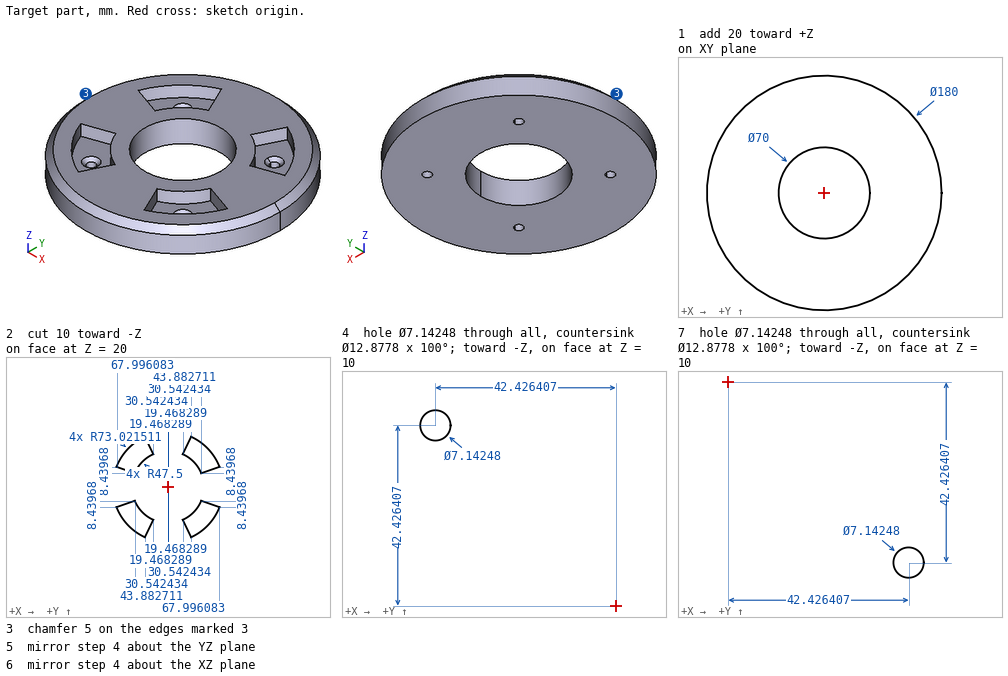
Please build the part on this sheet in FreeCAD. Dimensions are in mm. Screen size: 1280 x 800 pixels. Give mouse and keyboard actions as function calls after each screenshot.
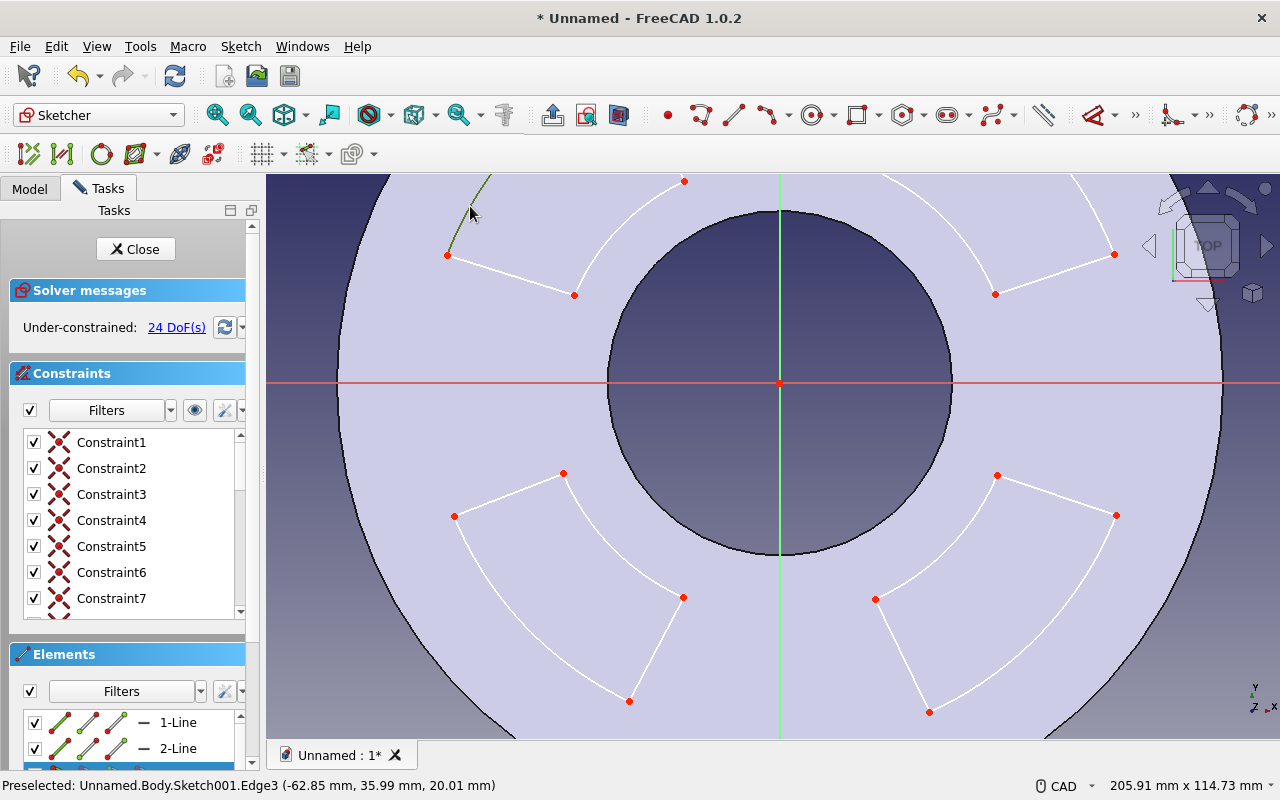
click(1091, 205)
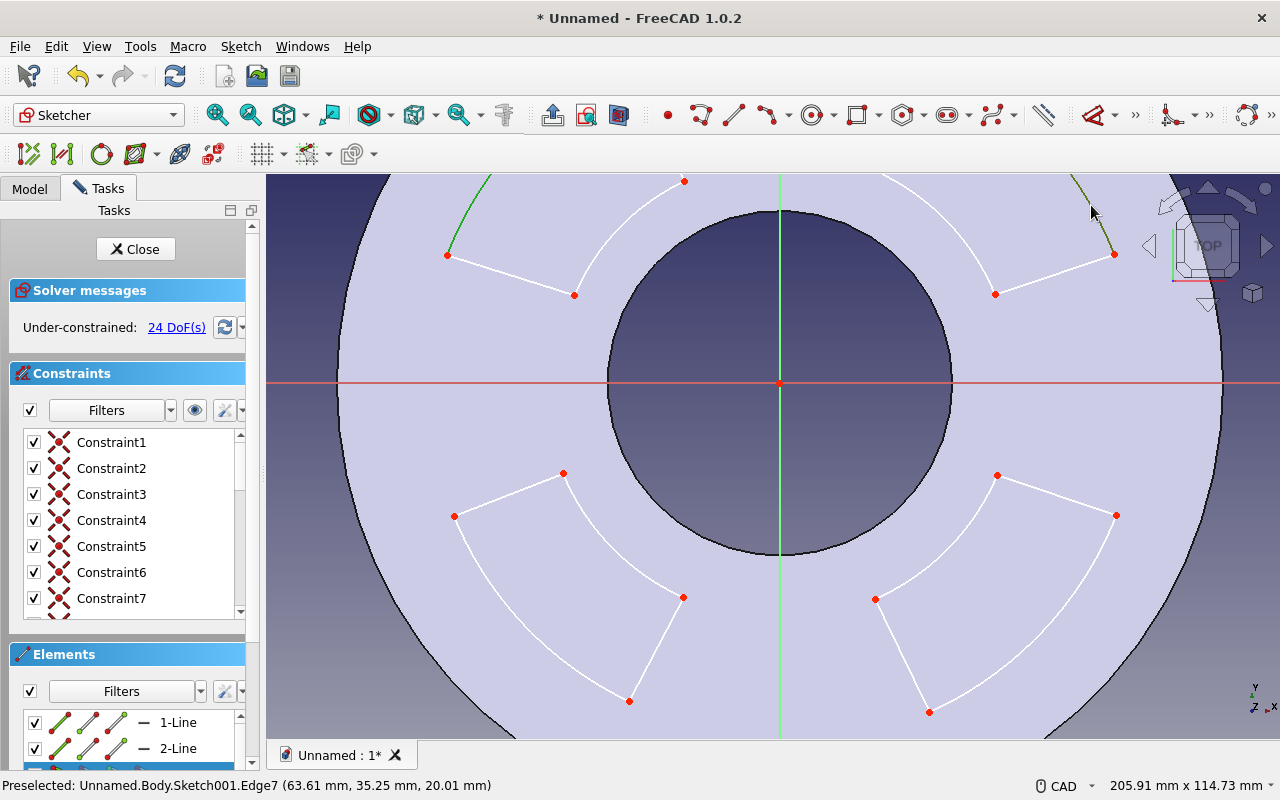
click(1001, 669)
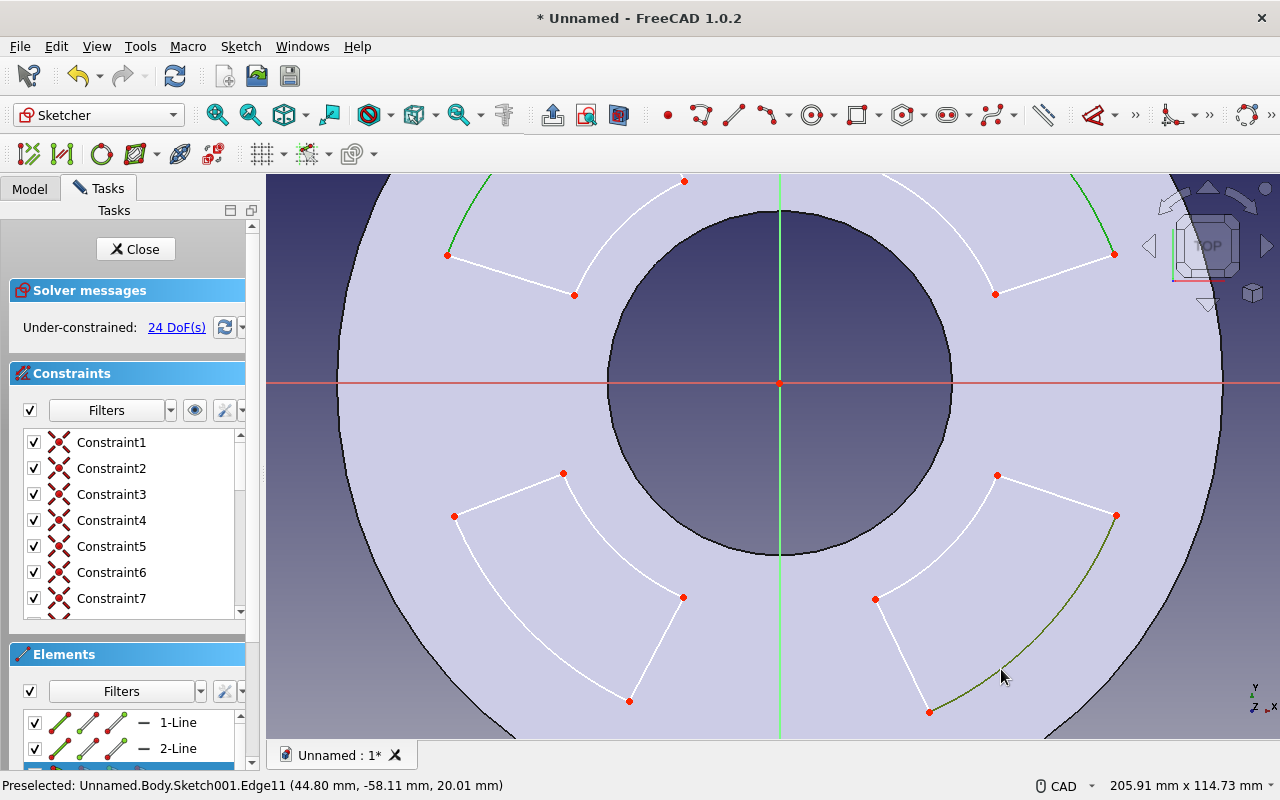
click(491, 585)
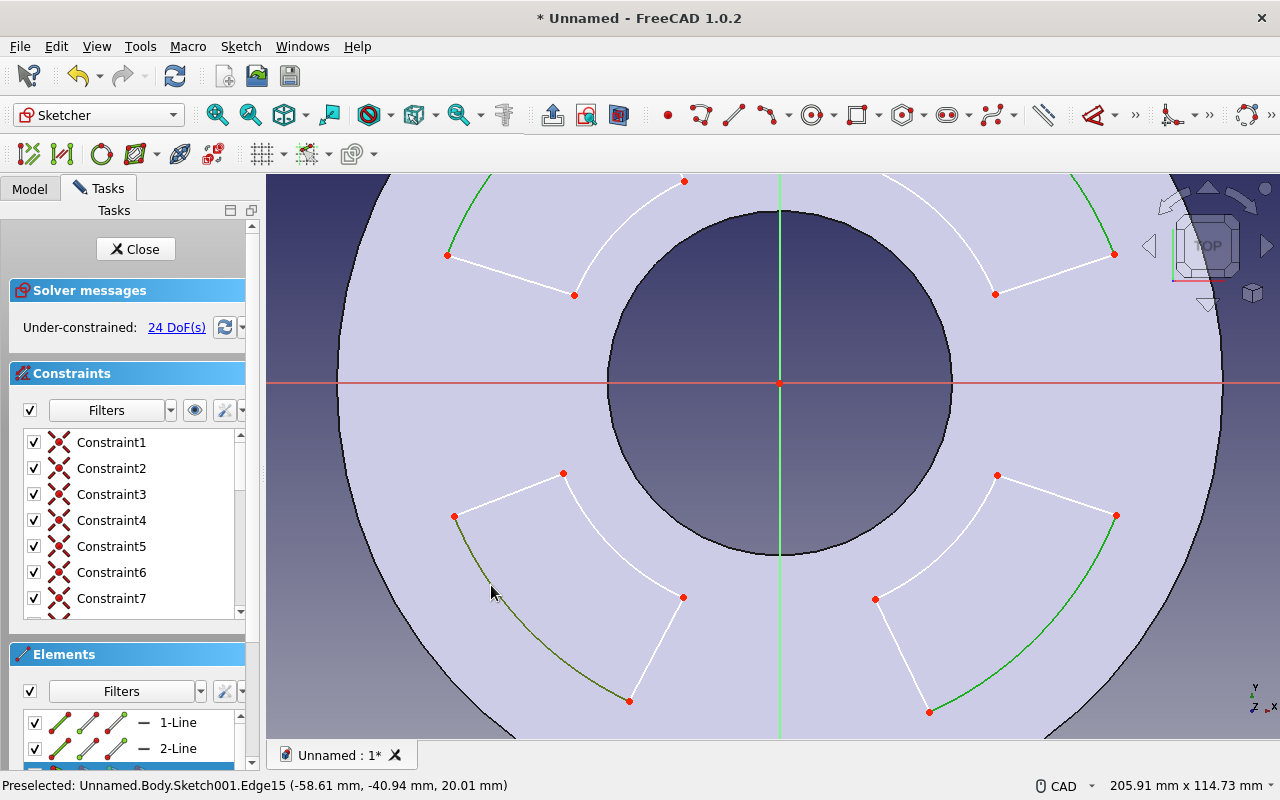
key(e)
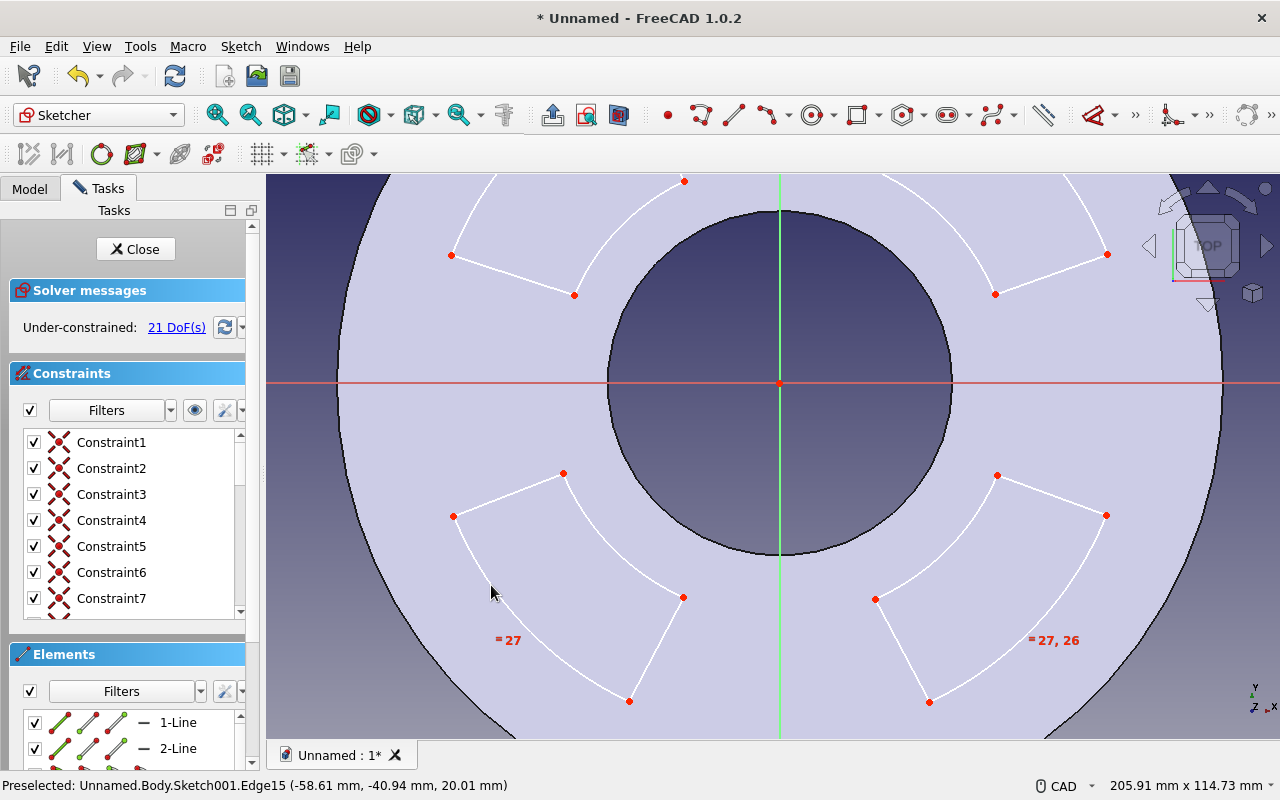
click(643, 207)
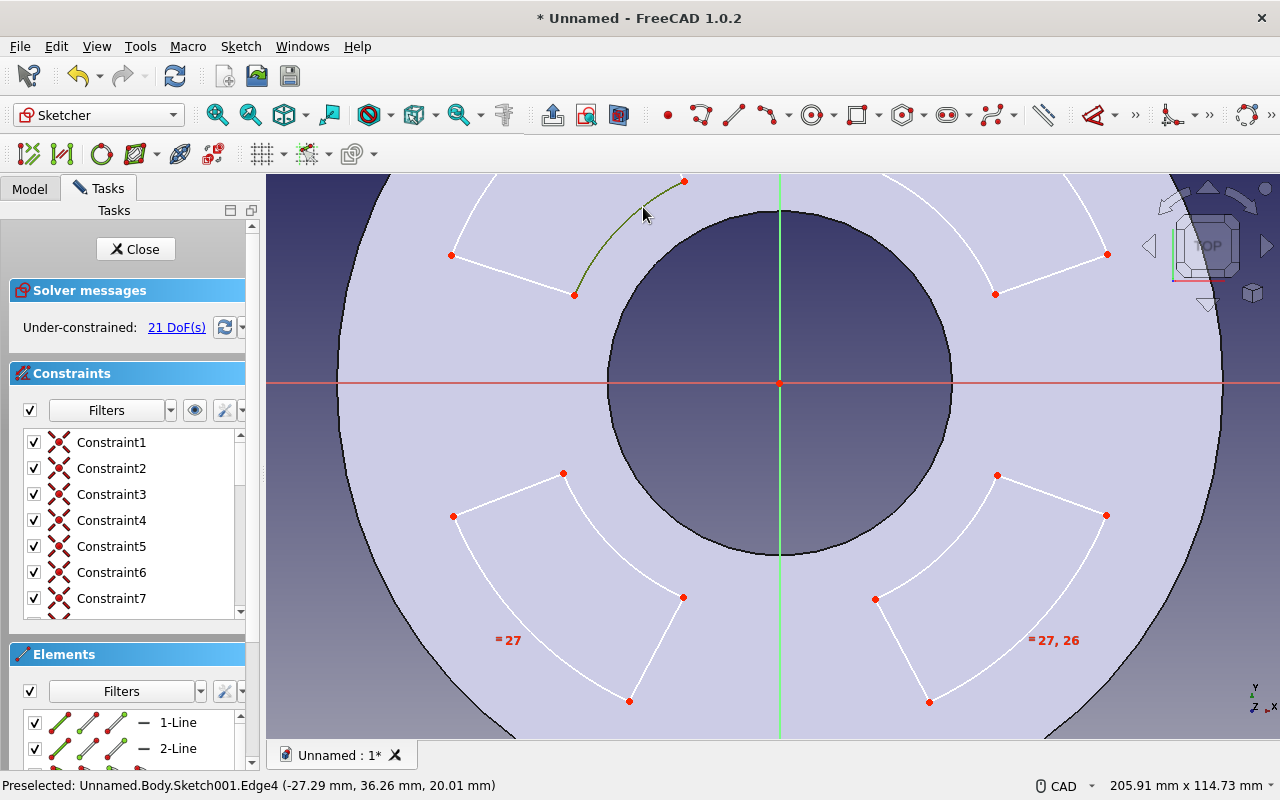
click(970, 248)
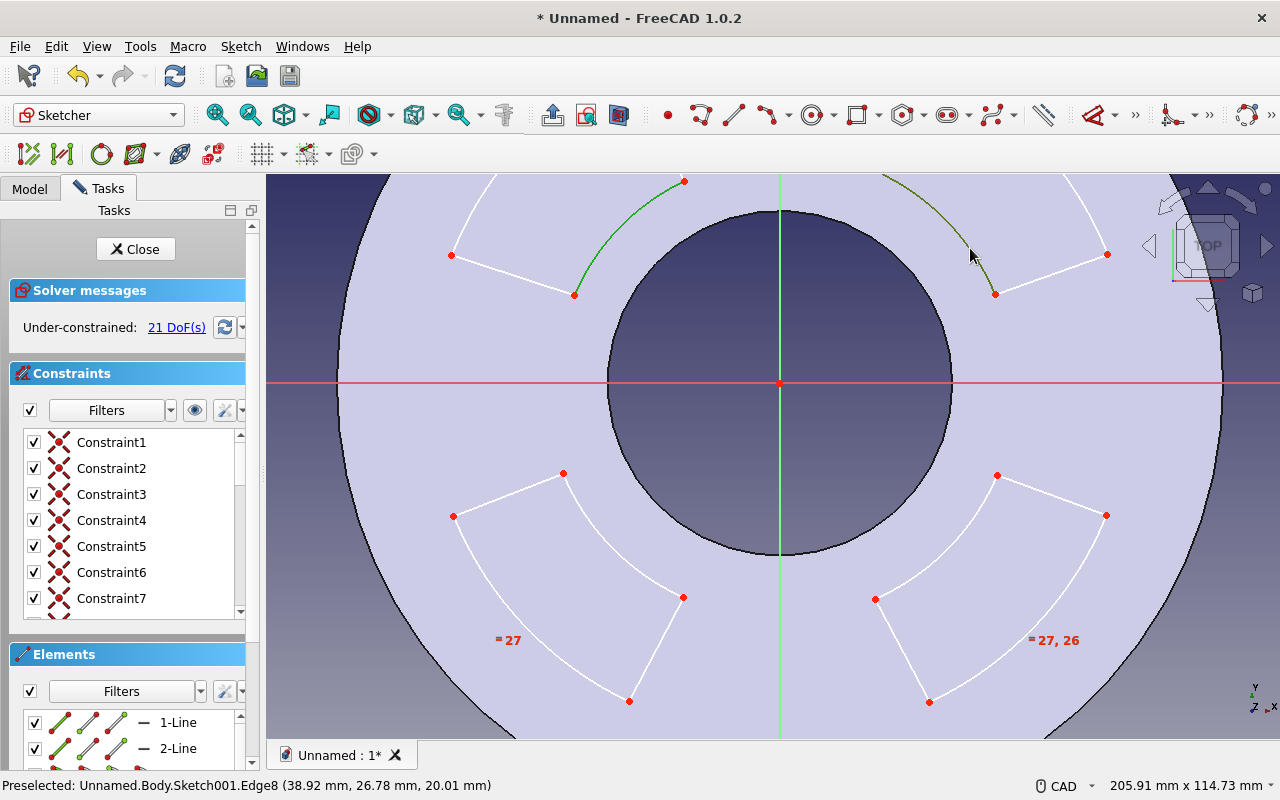
click(921, 572)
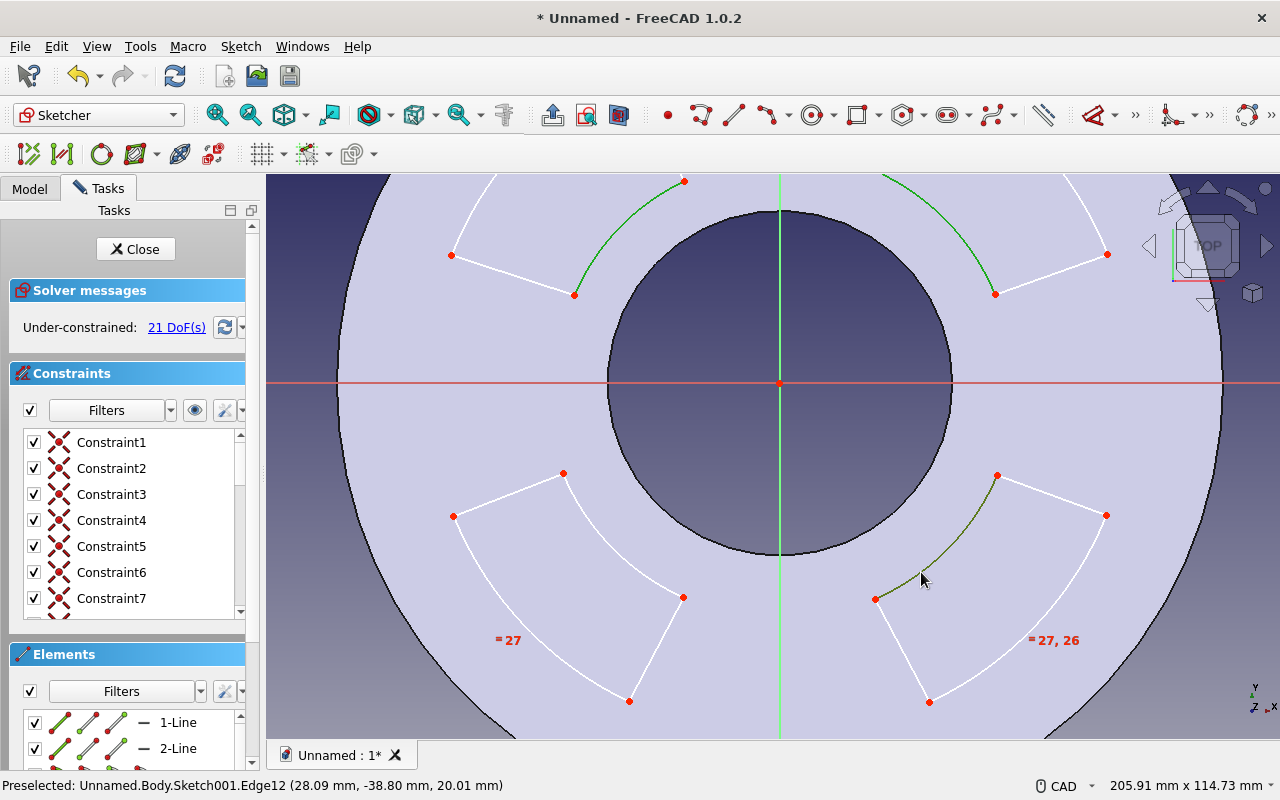
click(589, 520)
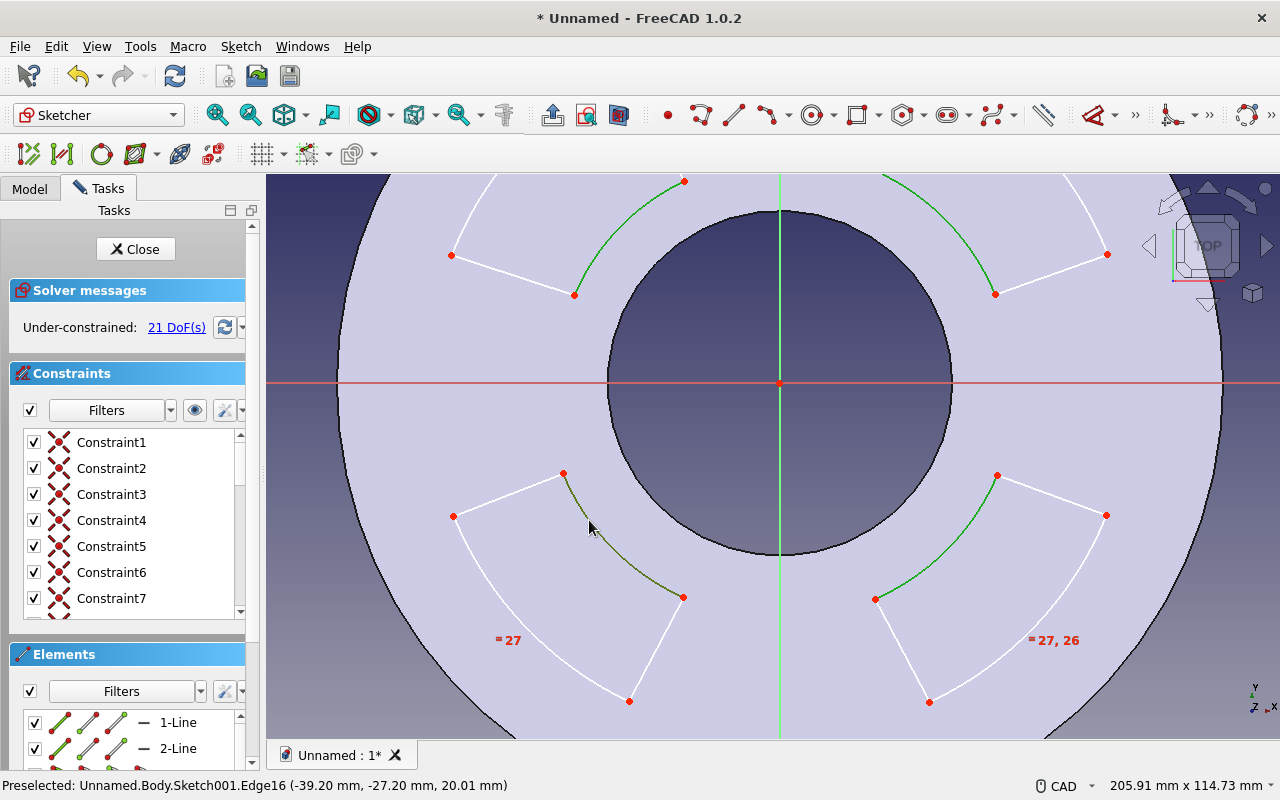
key(e)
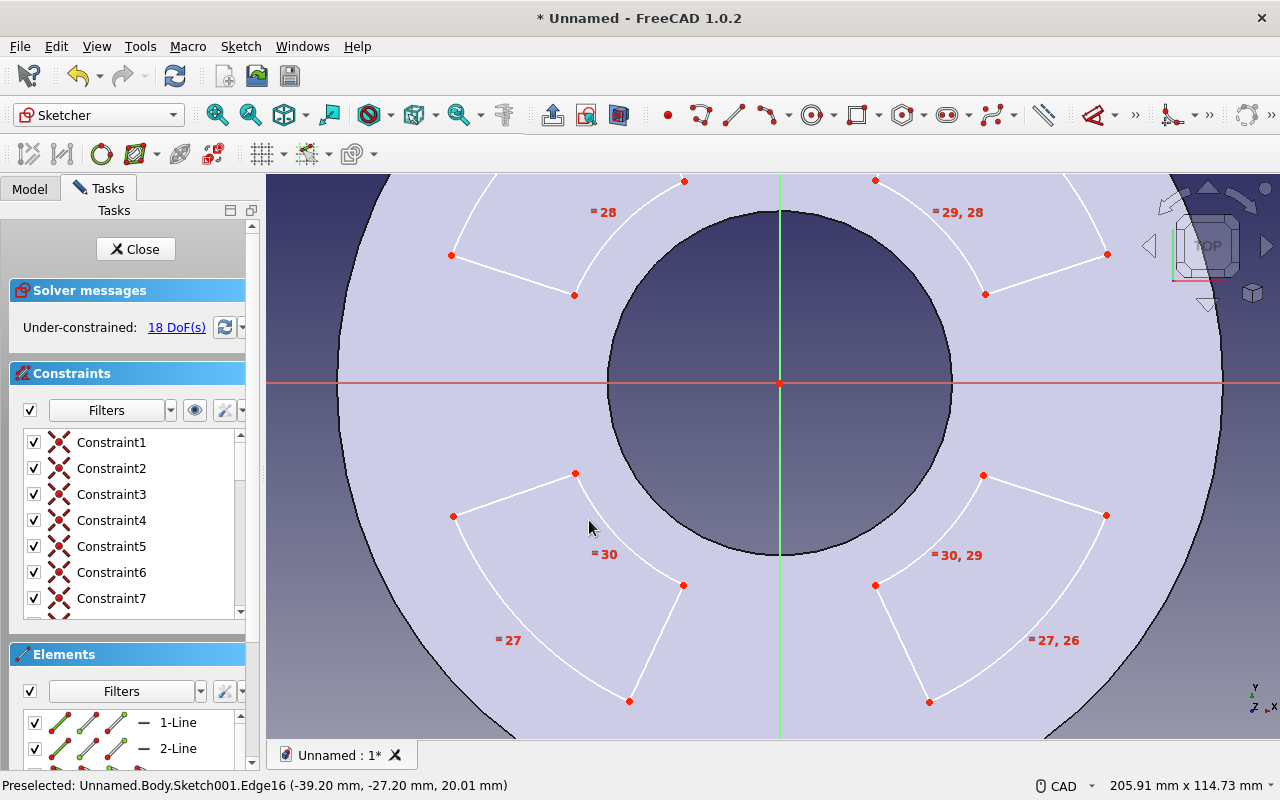
click(1092, 116)